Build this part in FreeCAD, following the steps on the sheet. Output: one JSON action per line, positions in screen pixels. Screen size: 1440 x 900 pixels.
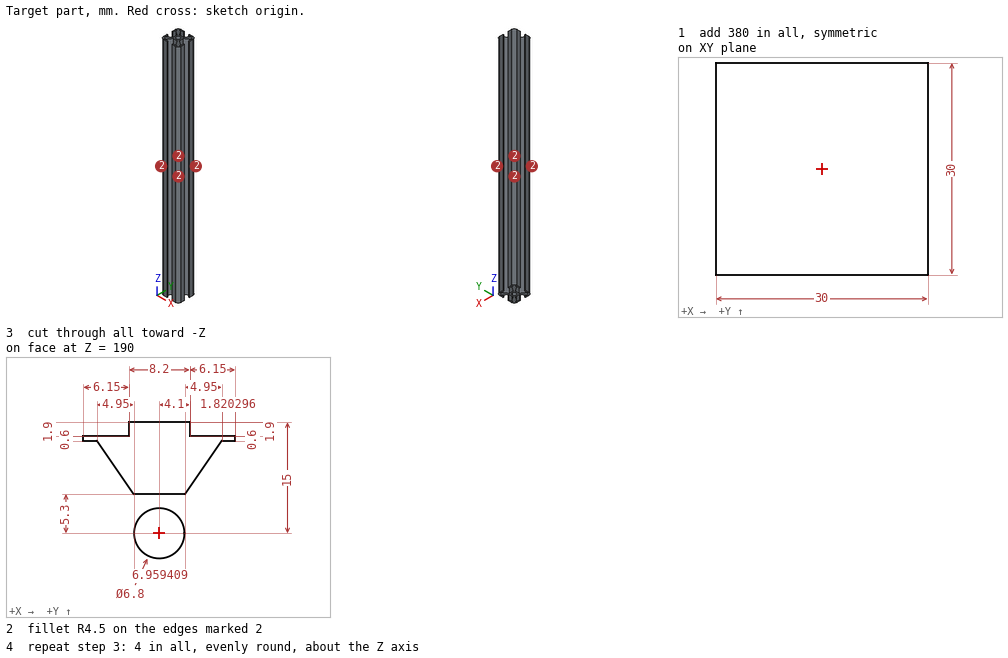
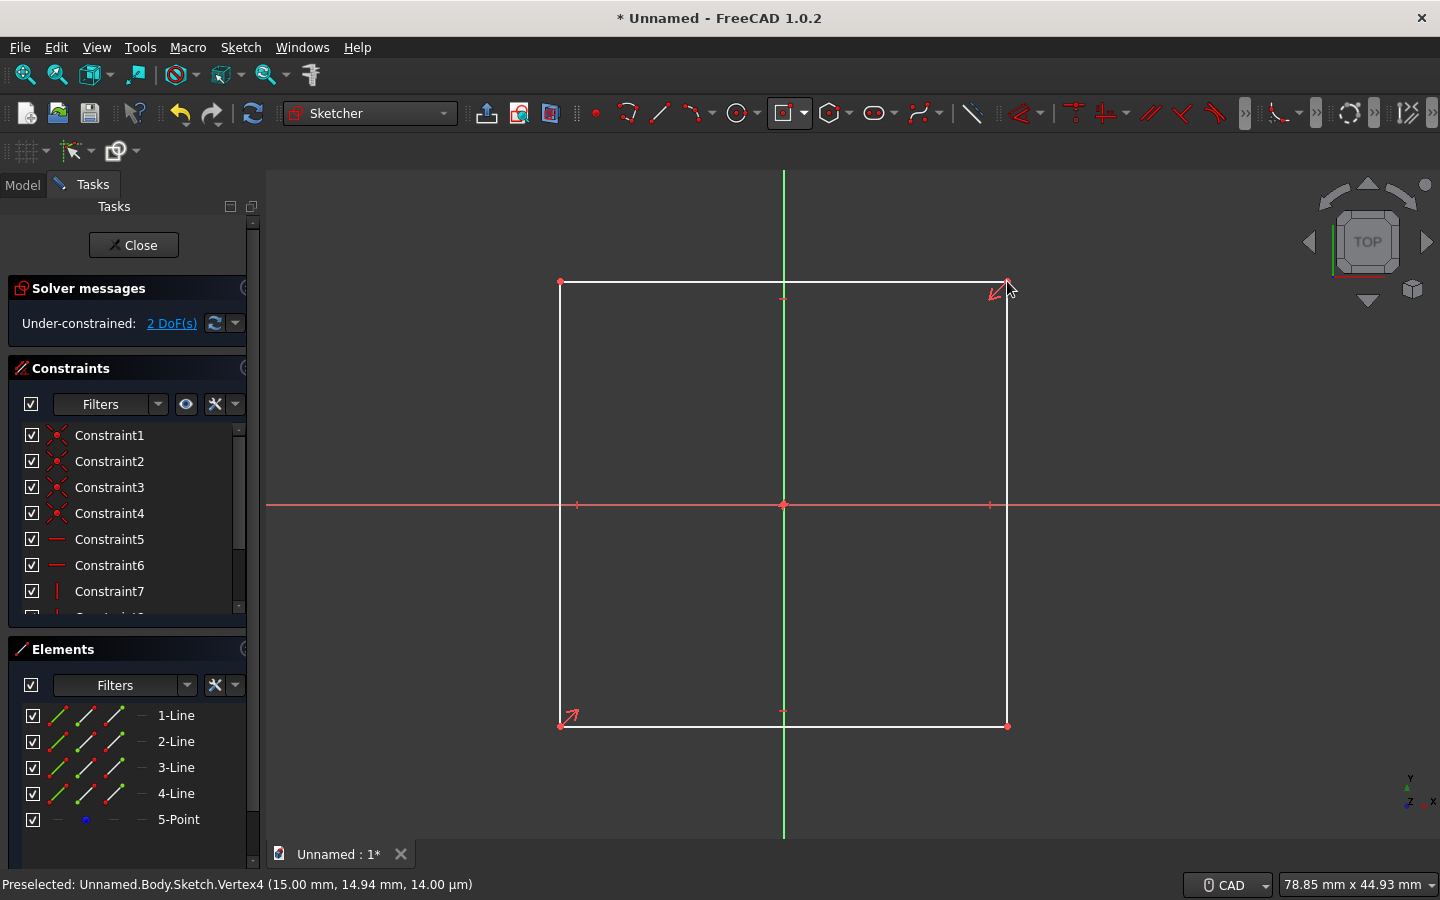
{"action": "left_click", "coordinate": [1020, 114]}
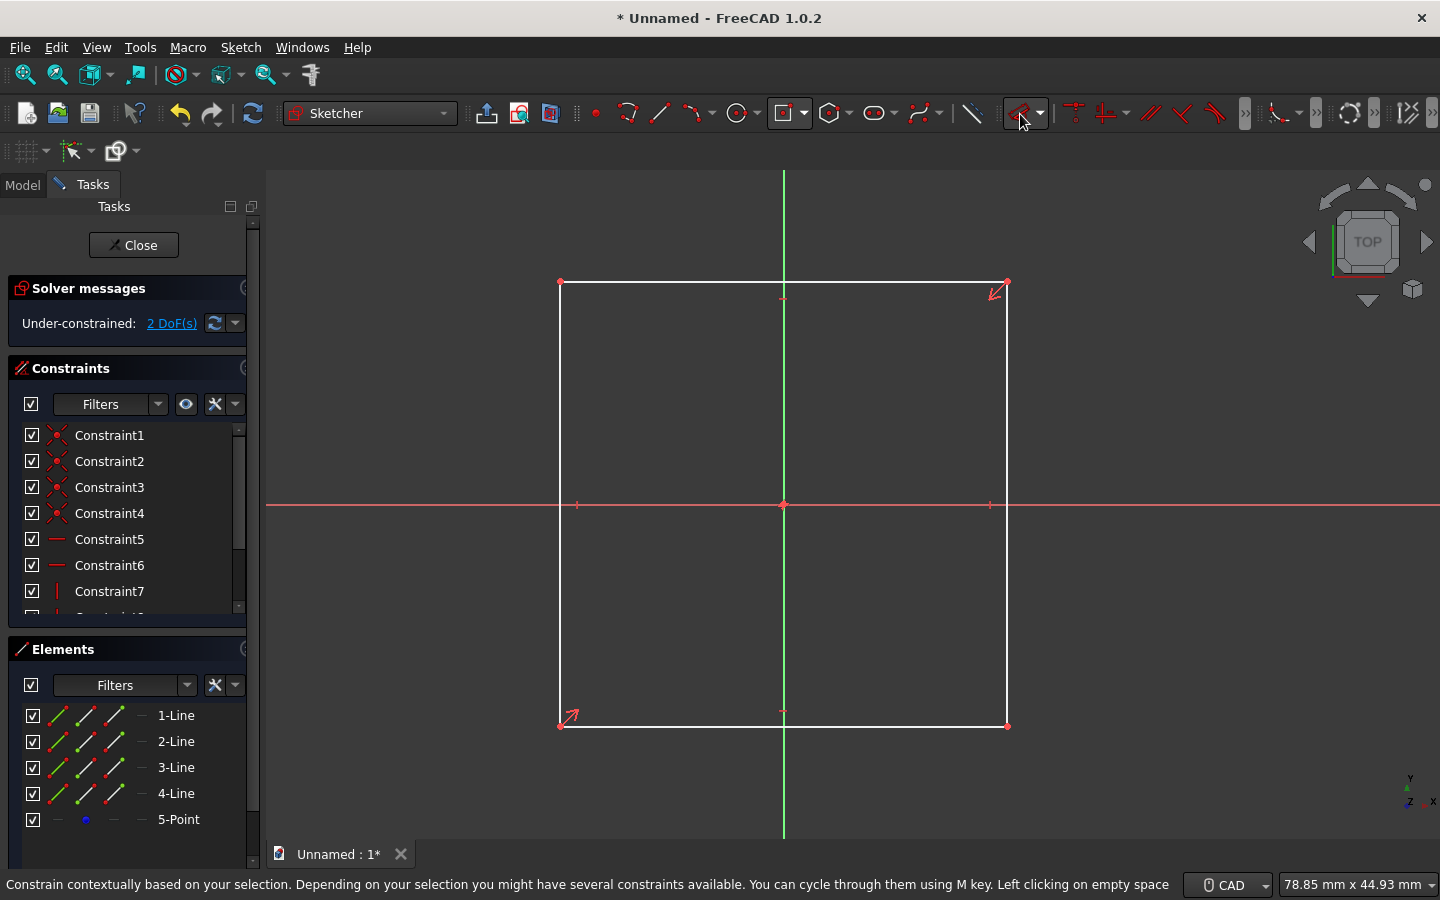
{"action": "left_click", "coordinate": [694, 727]}
{"action": "left_click", "coordinate": [681, 761]}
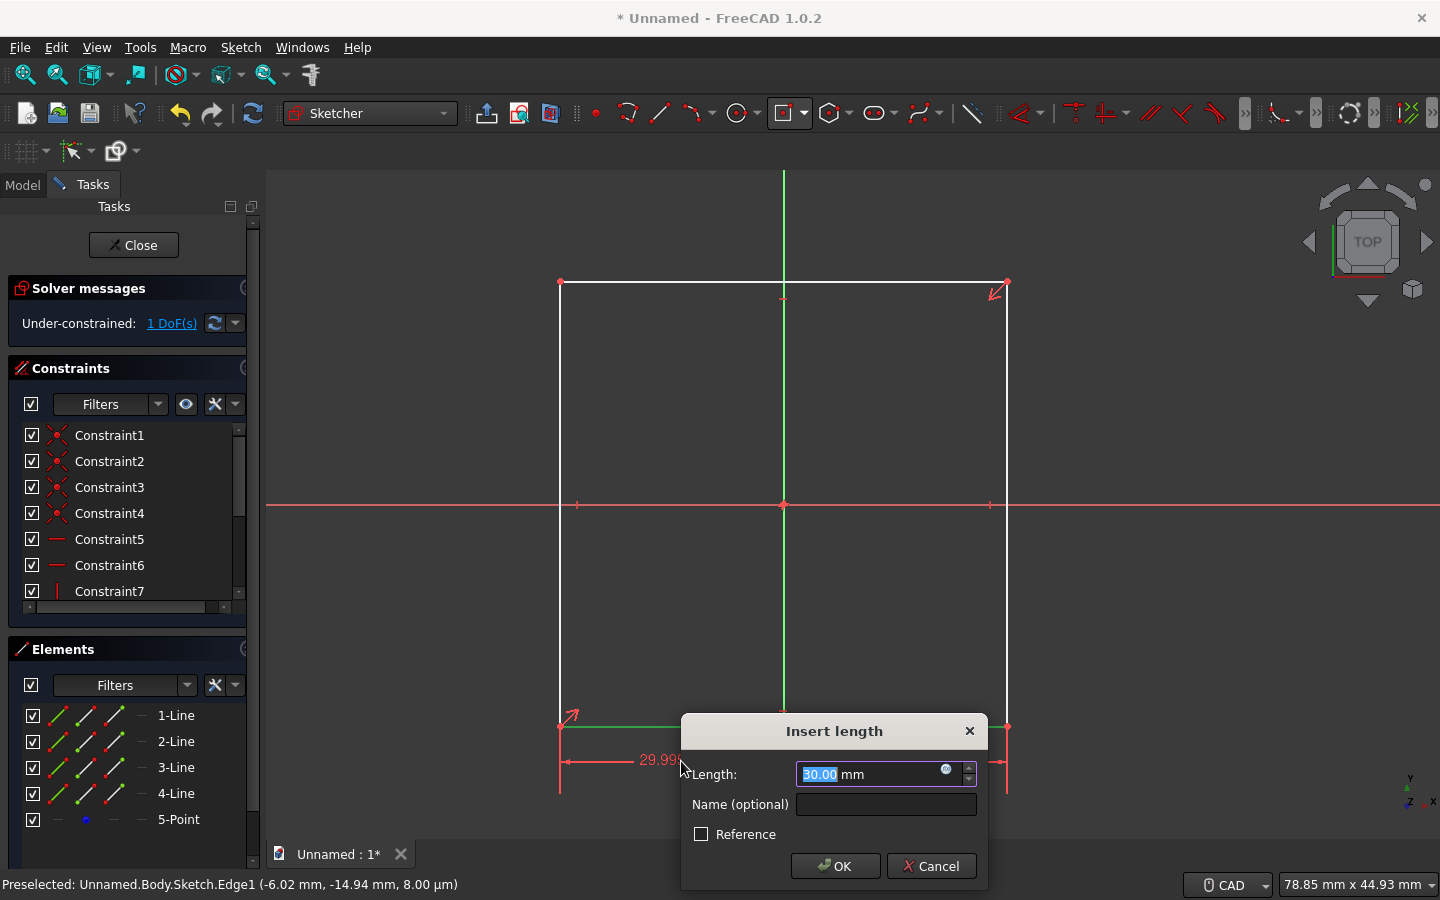
{"action": "type", "text": "30"}
{"action": "key", "text": "Return"}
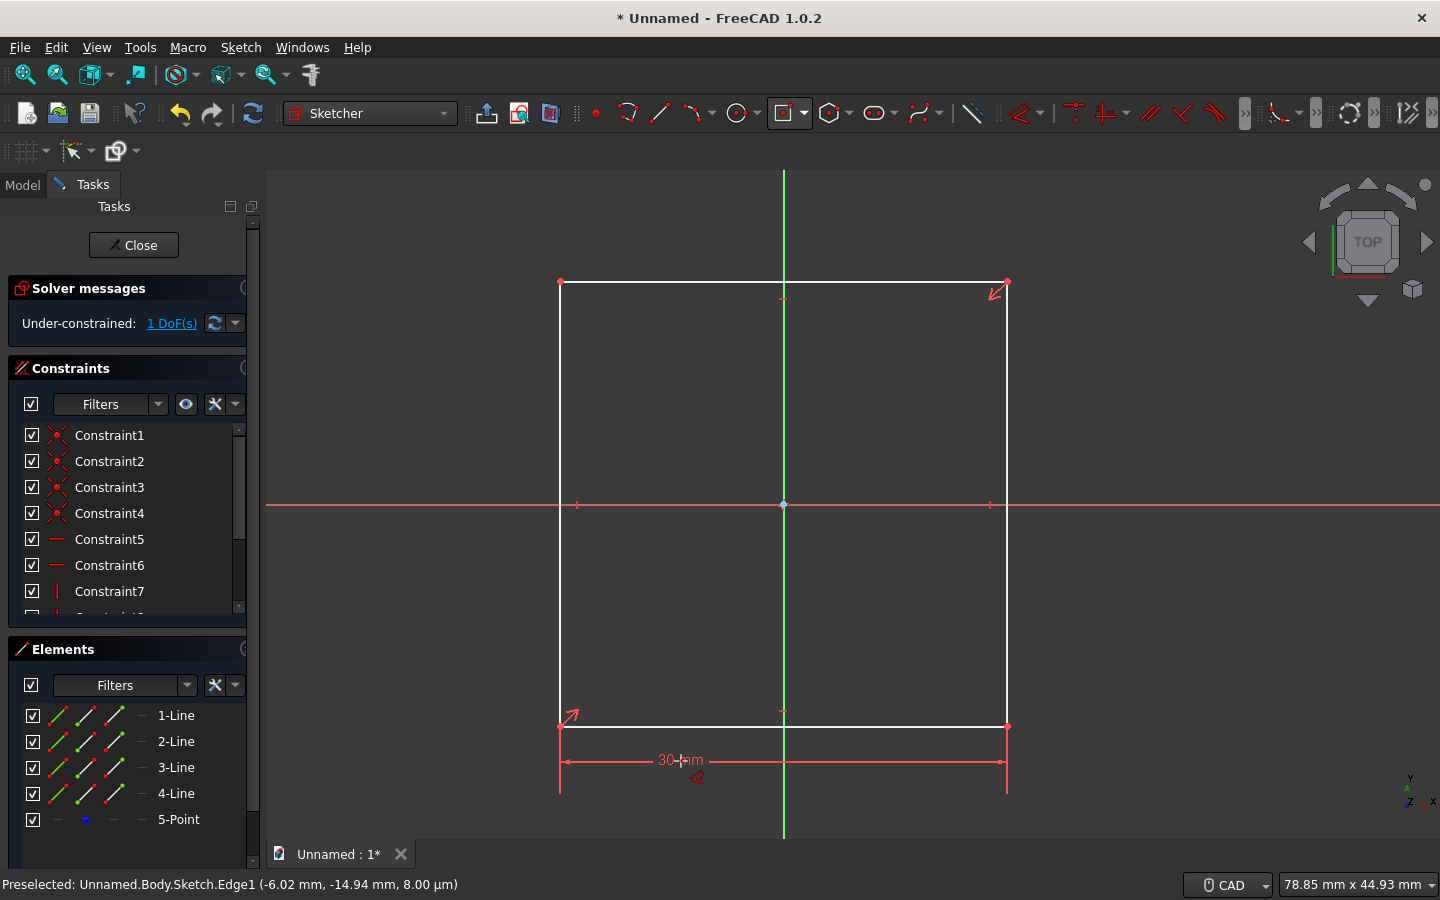
{"action": "left_click", "coordinate": [1007, 593]}
{"action": "left_click", "coordinate": [1041, 402]}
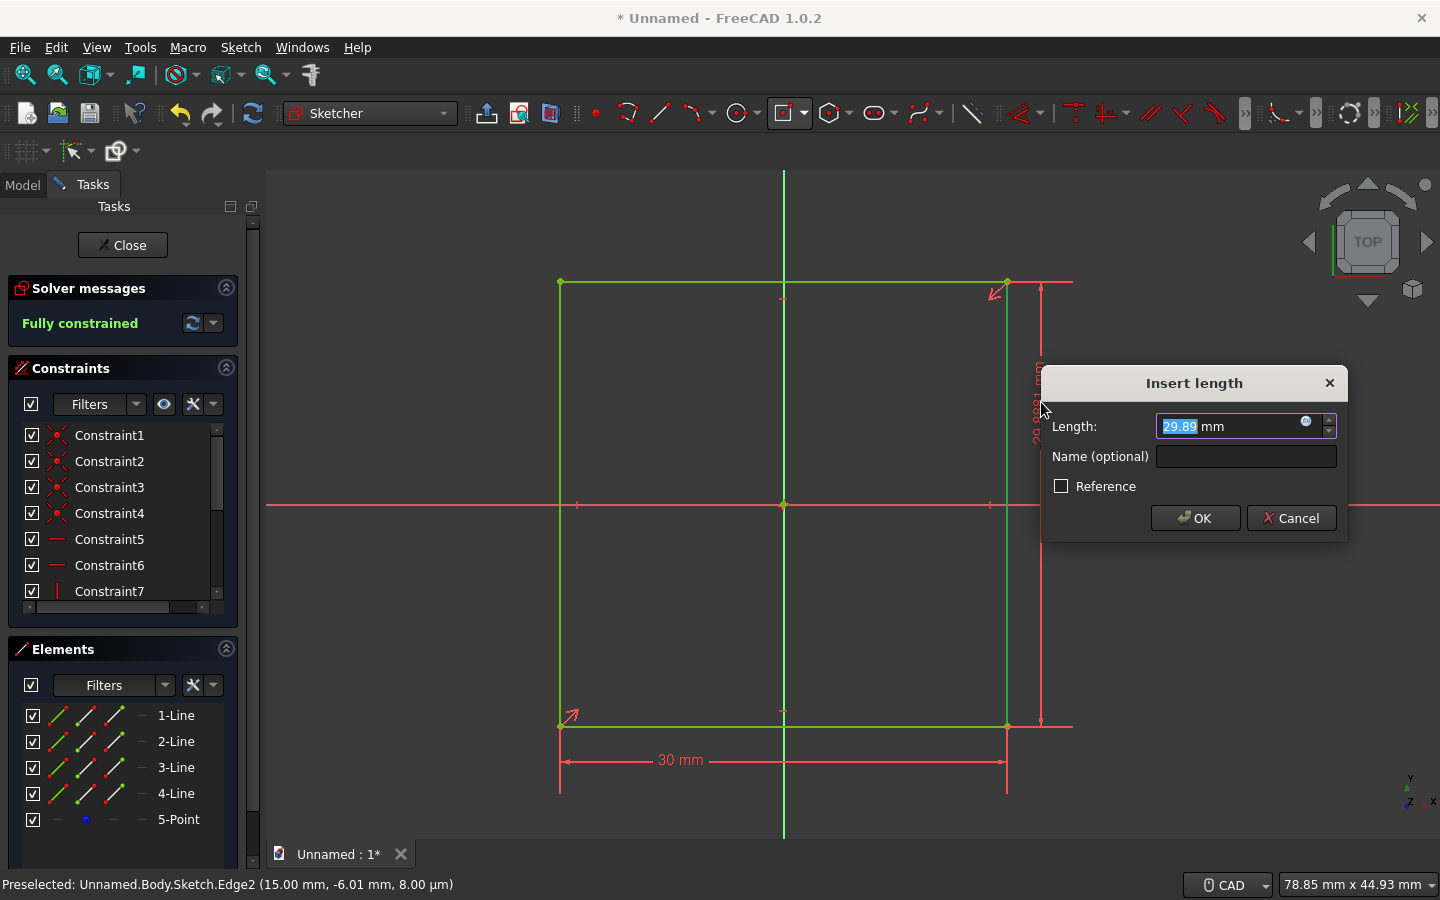
{"action": "type", "text": "30"}
{"action": "key", "text": "Return"}
{"action": "key", "text": "Escape"}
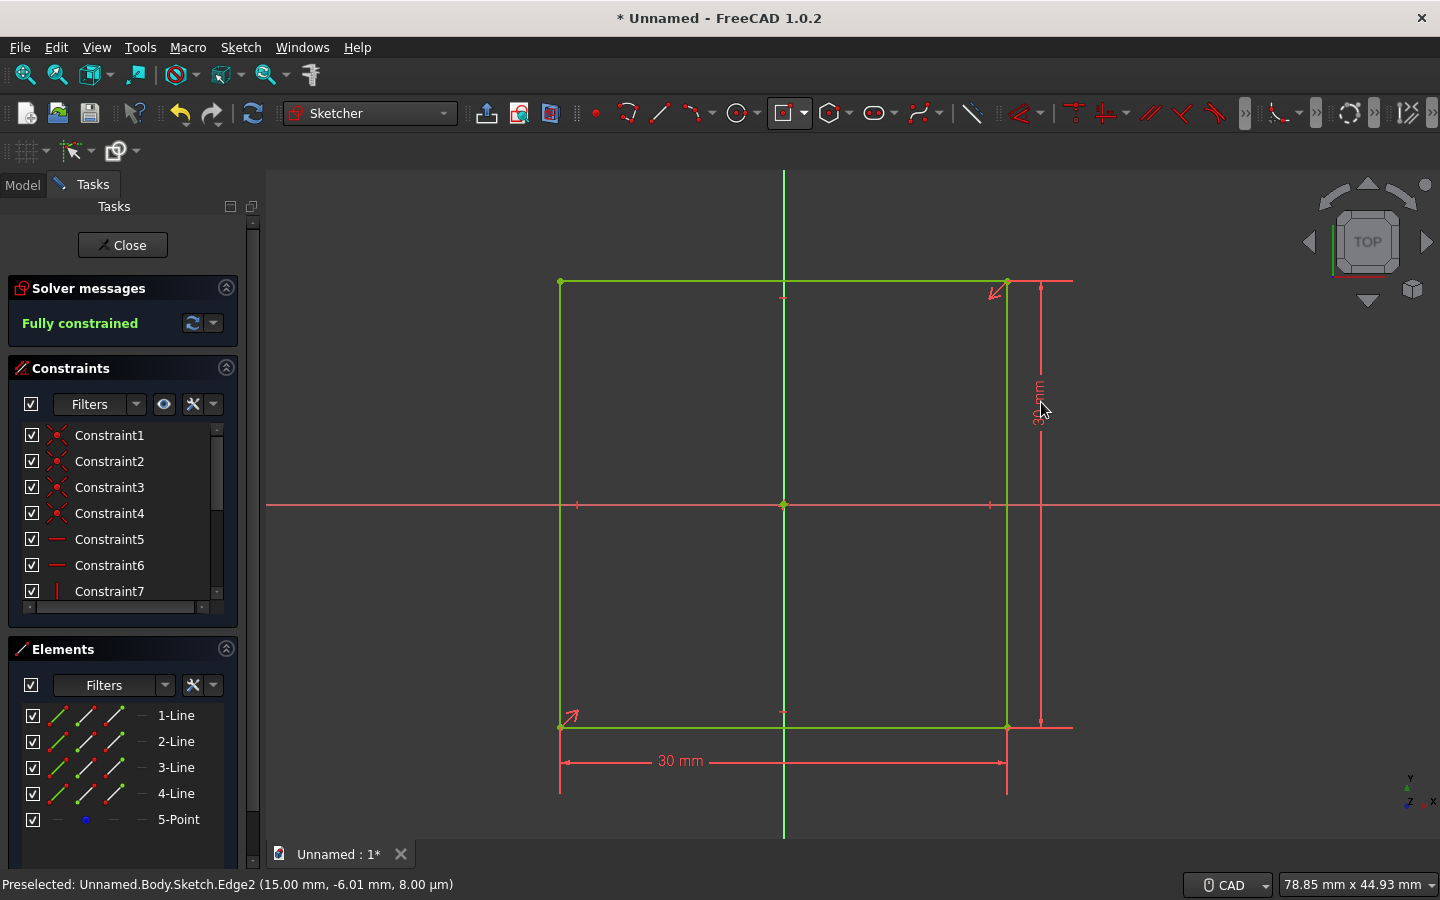
{"action": "left_click", "coordinate": [123, 245]}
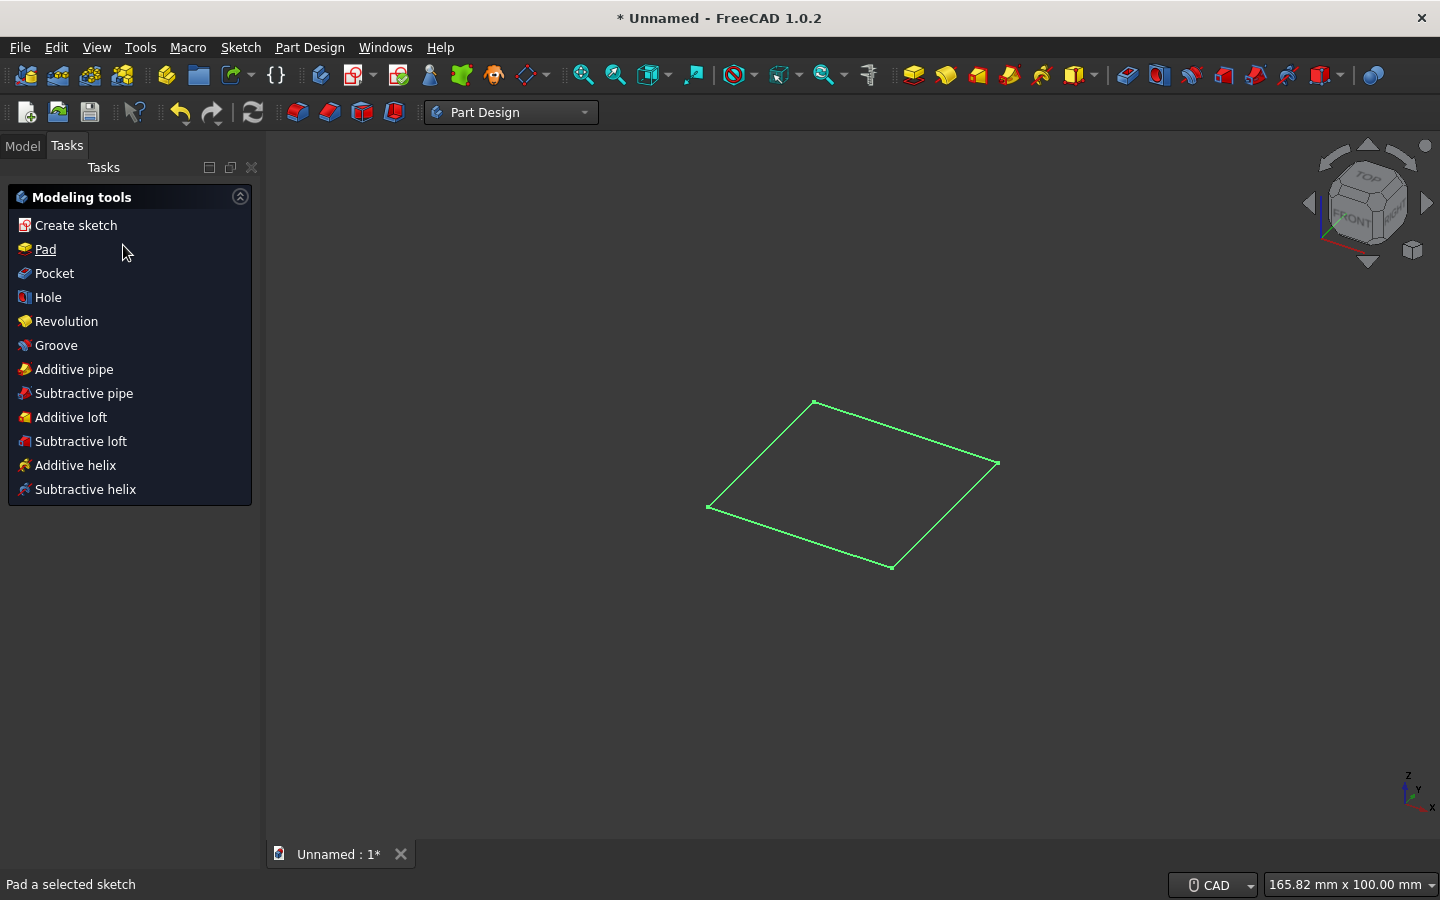
{"action": "left_click", "coordinate": [914, 76]}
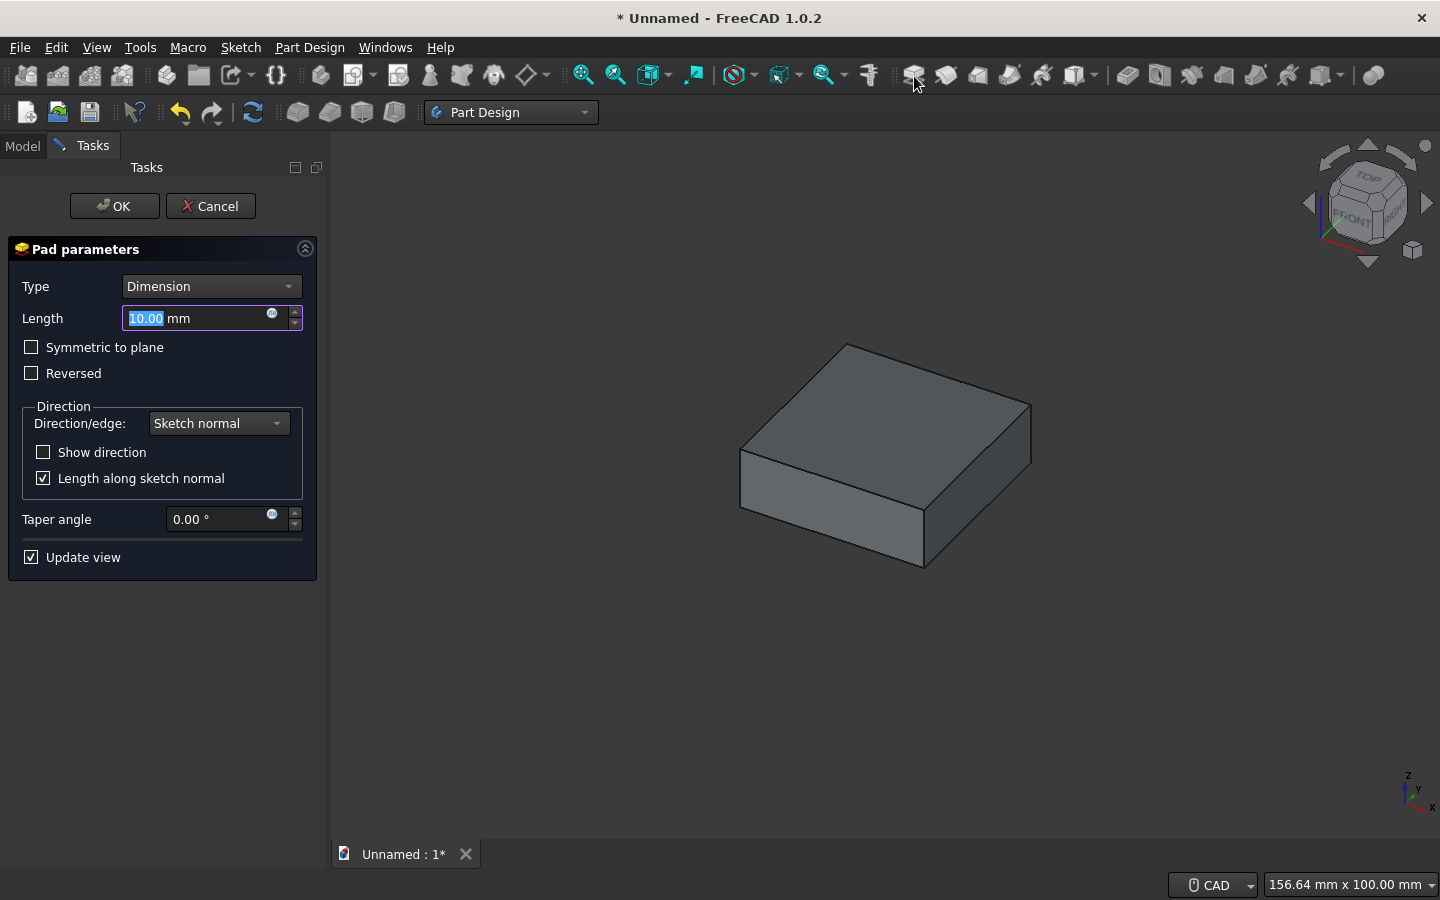
{"action": "type", "text": "380"}
{"action": "key", "text": "Tab"}